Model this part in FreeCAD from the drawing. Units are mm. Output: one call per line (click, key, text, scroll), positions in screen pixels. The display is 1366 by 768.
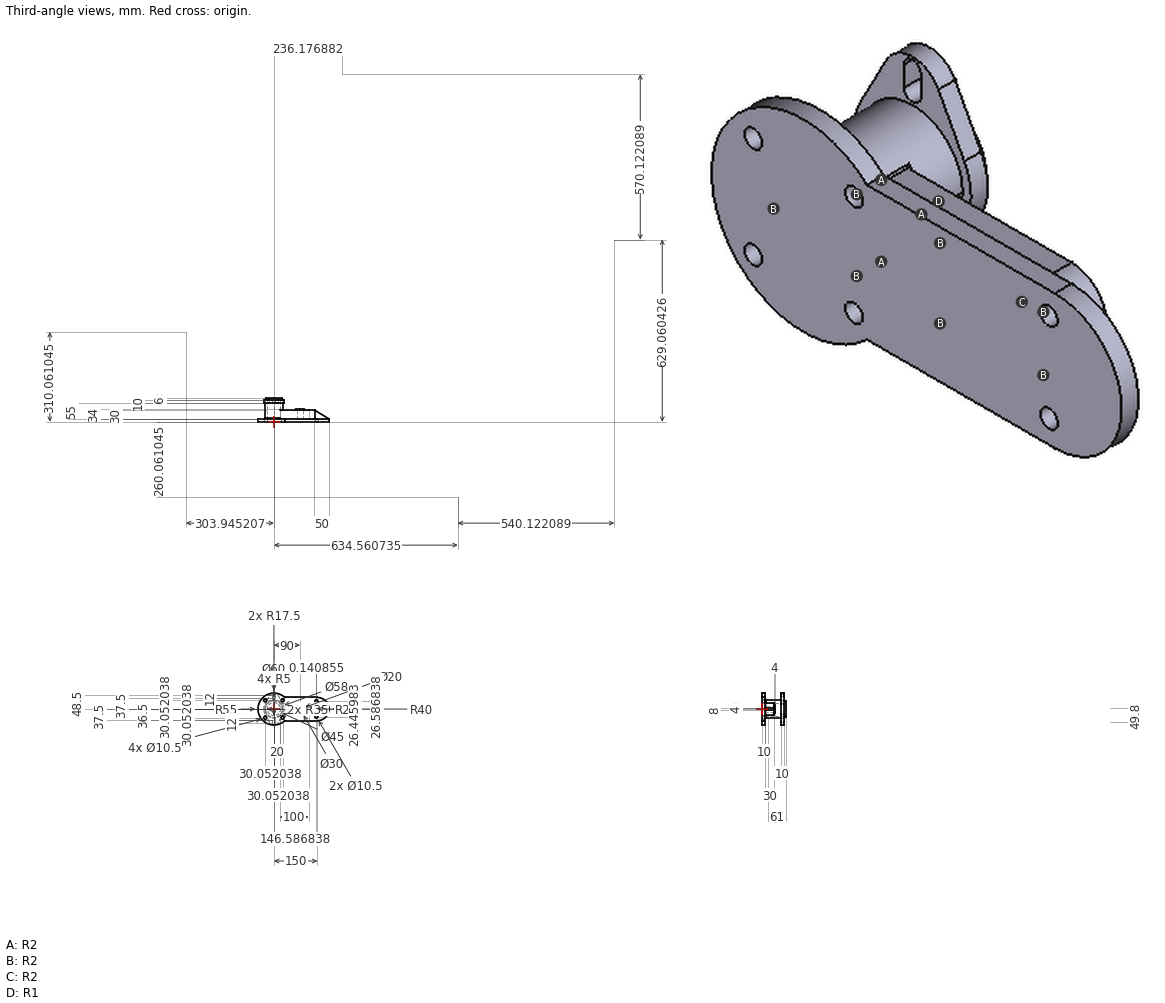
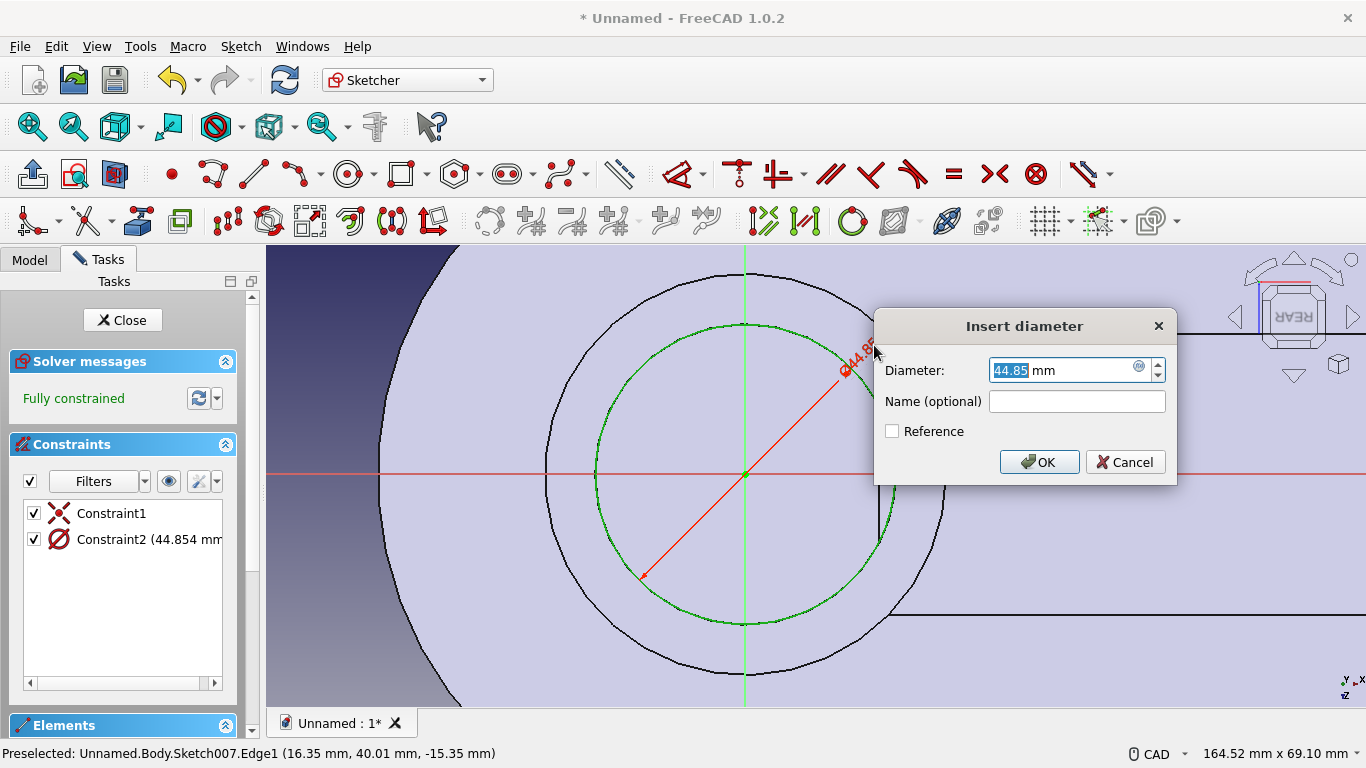
text(45)
key(Return)
key(Escape)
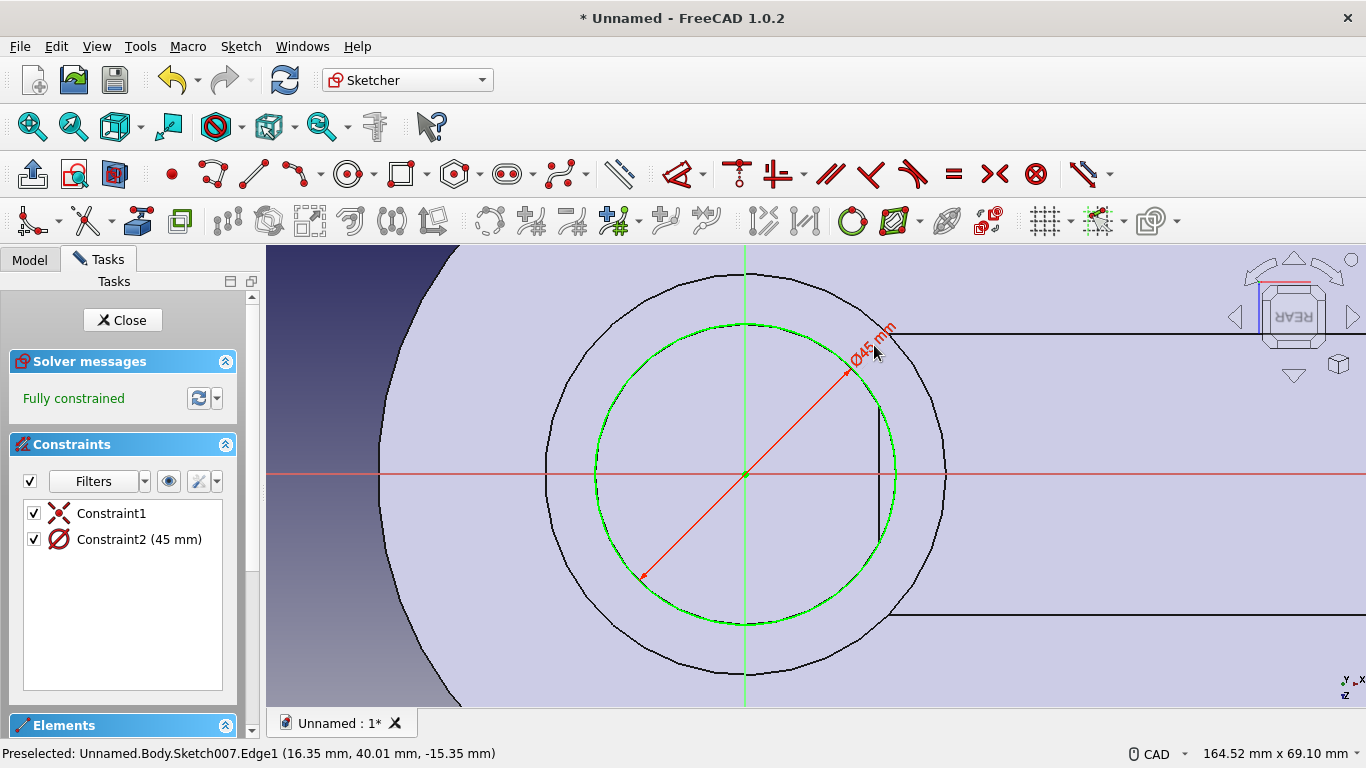
click(123, 320)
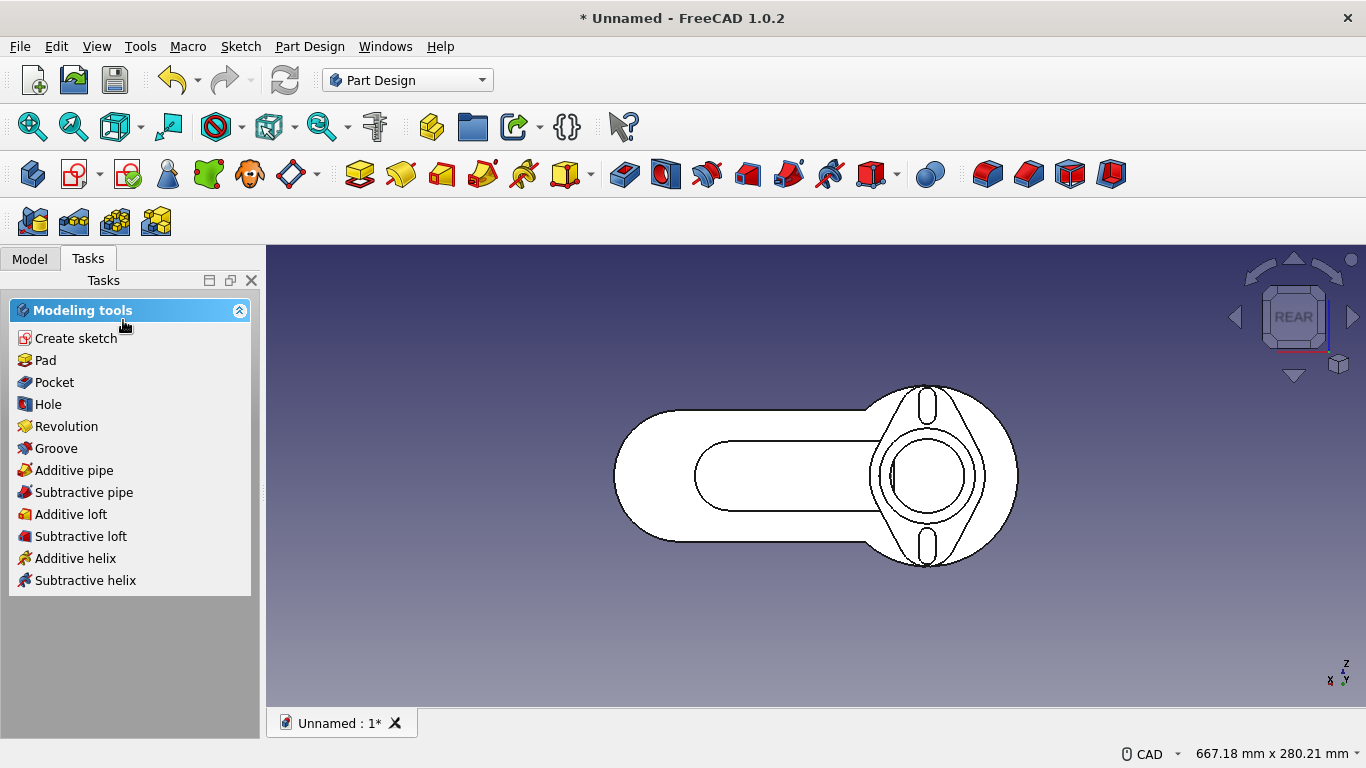
click(625, 174)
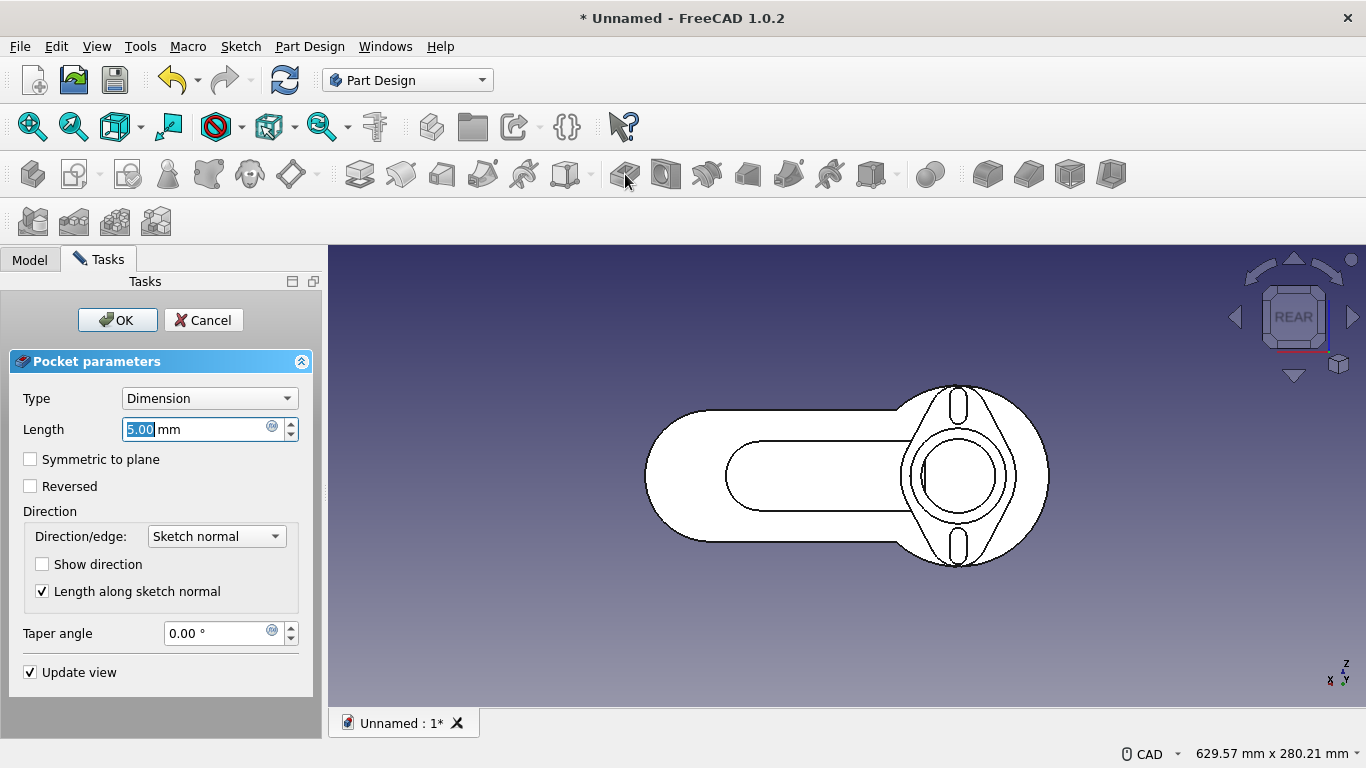
text(30)
key(Tab)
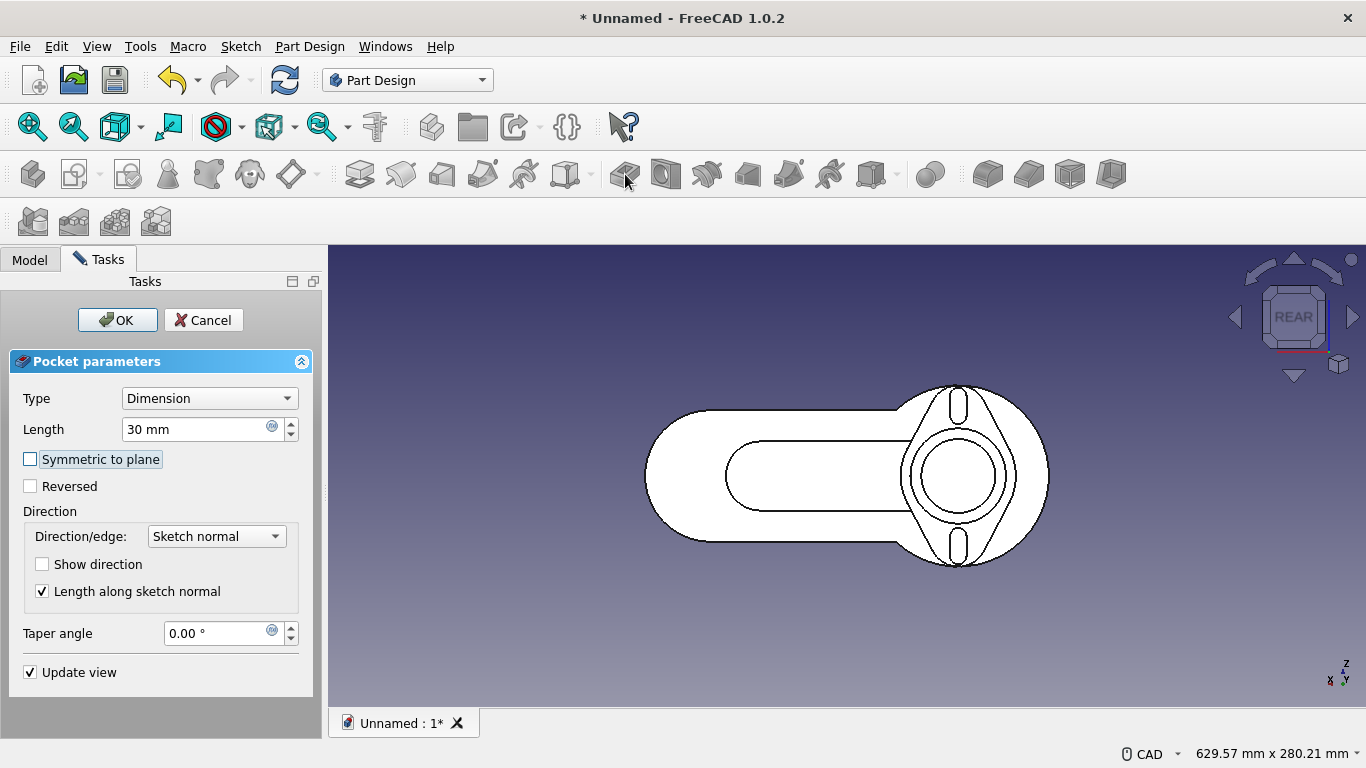
click(118, 320)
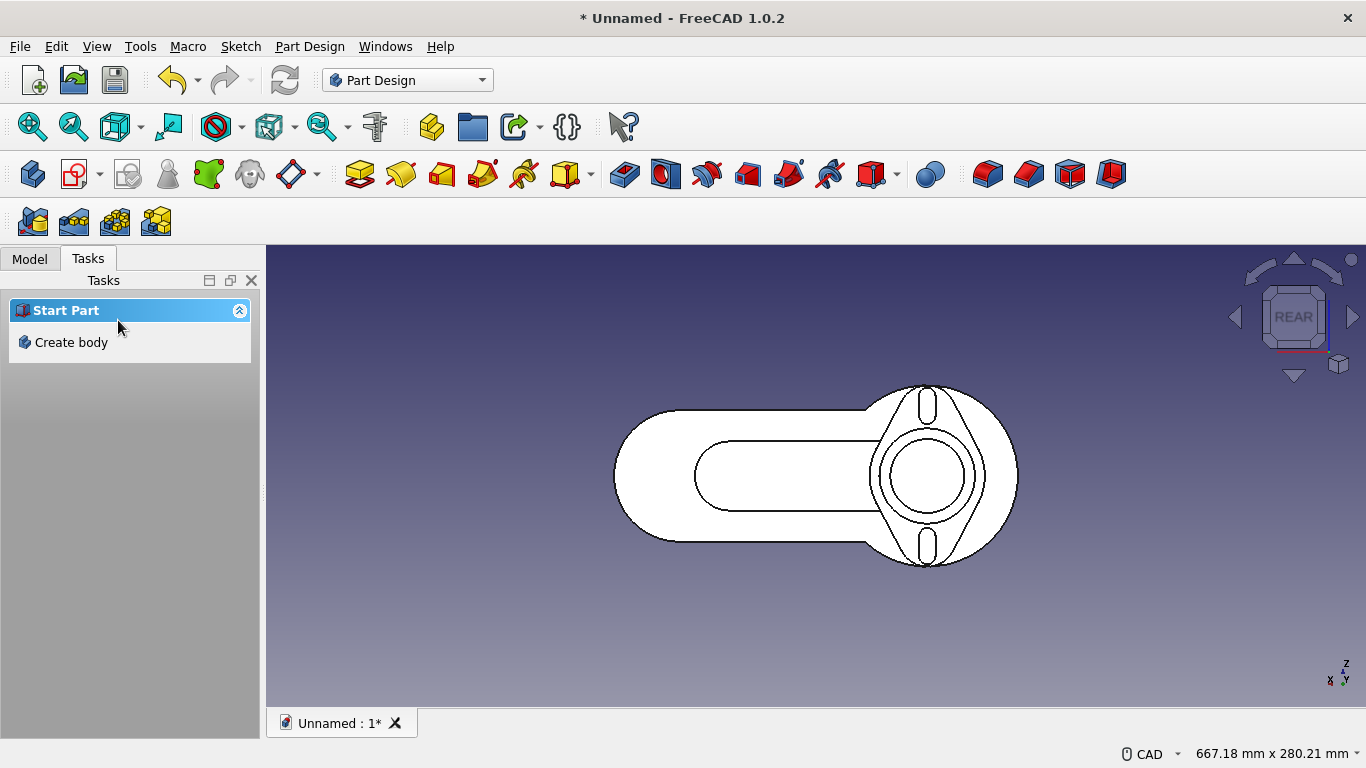
key(v)
key(f)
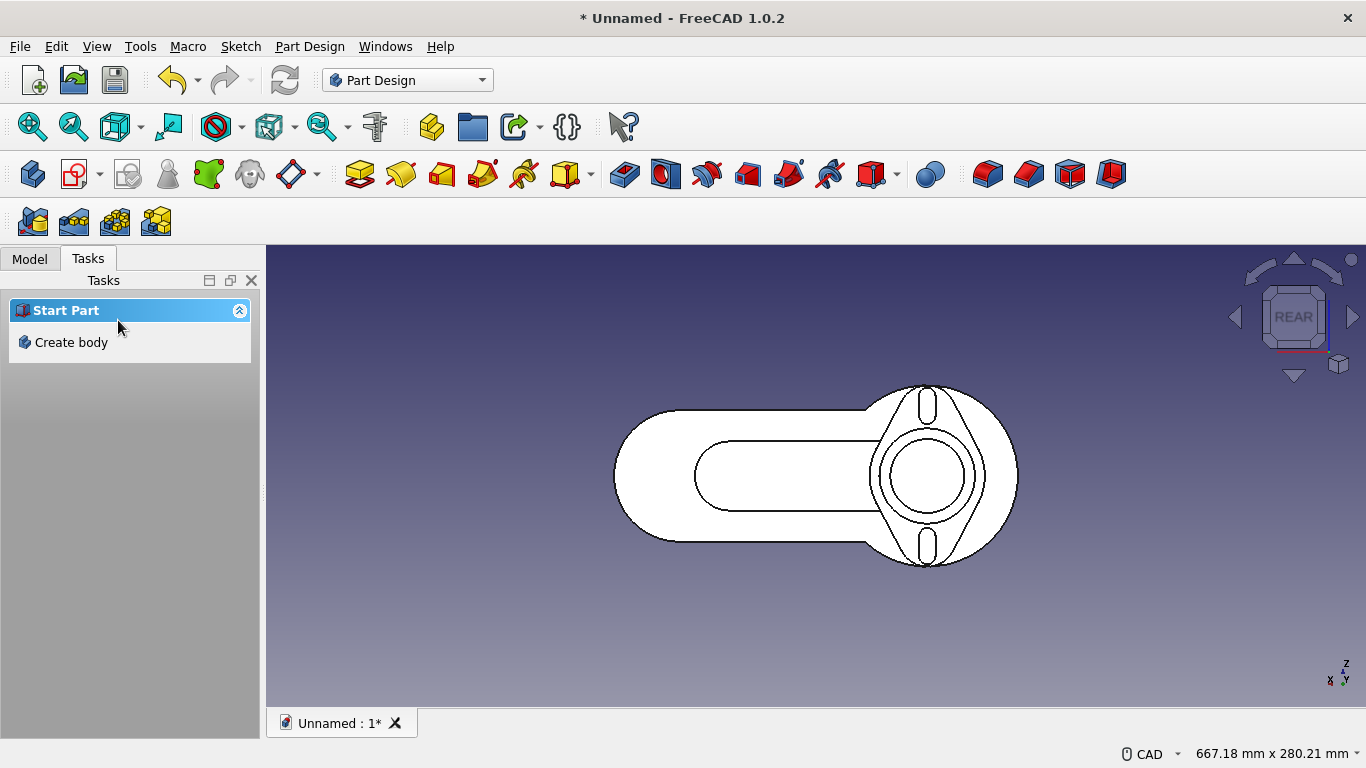
click(737, 475)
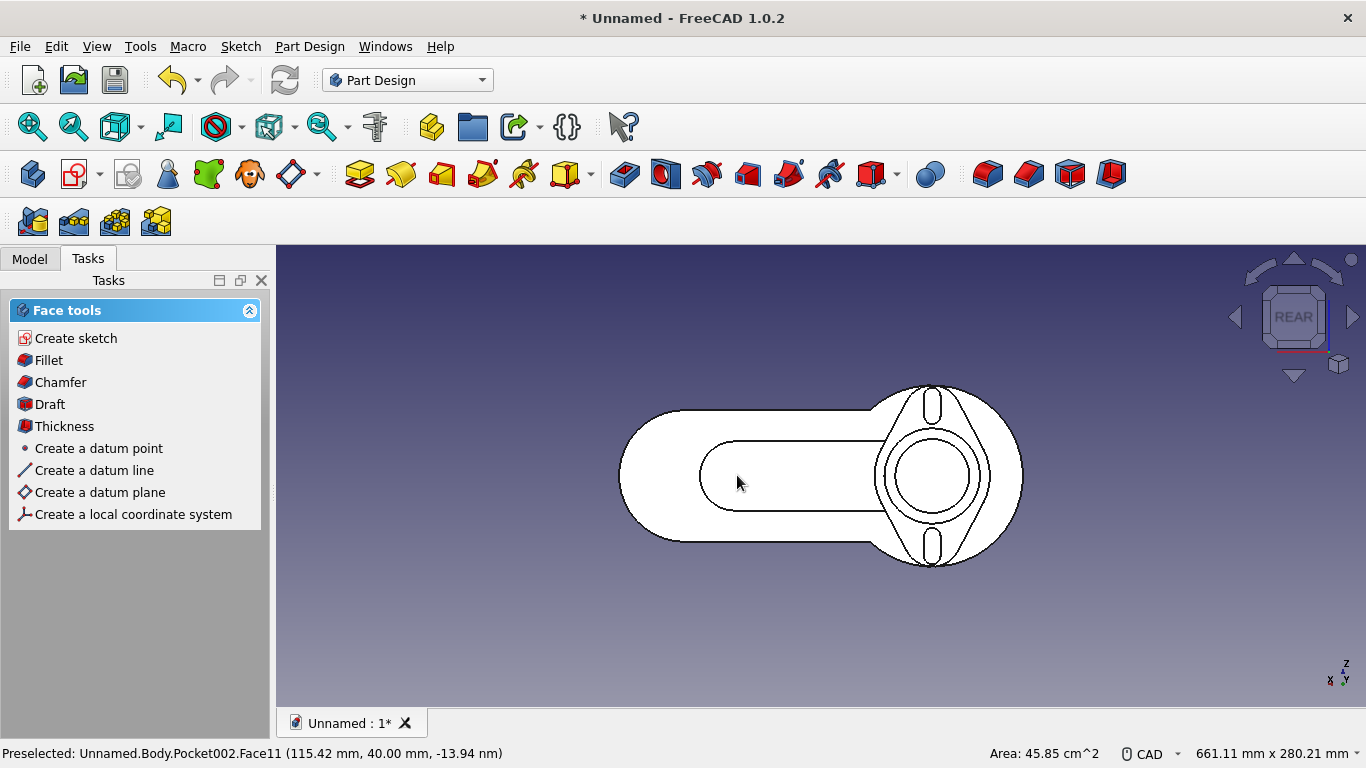
click(74, 174)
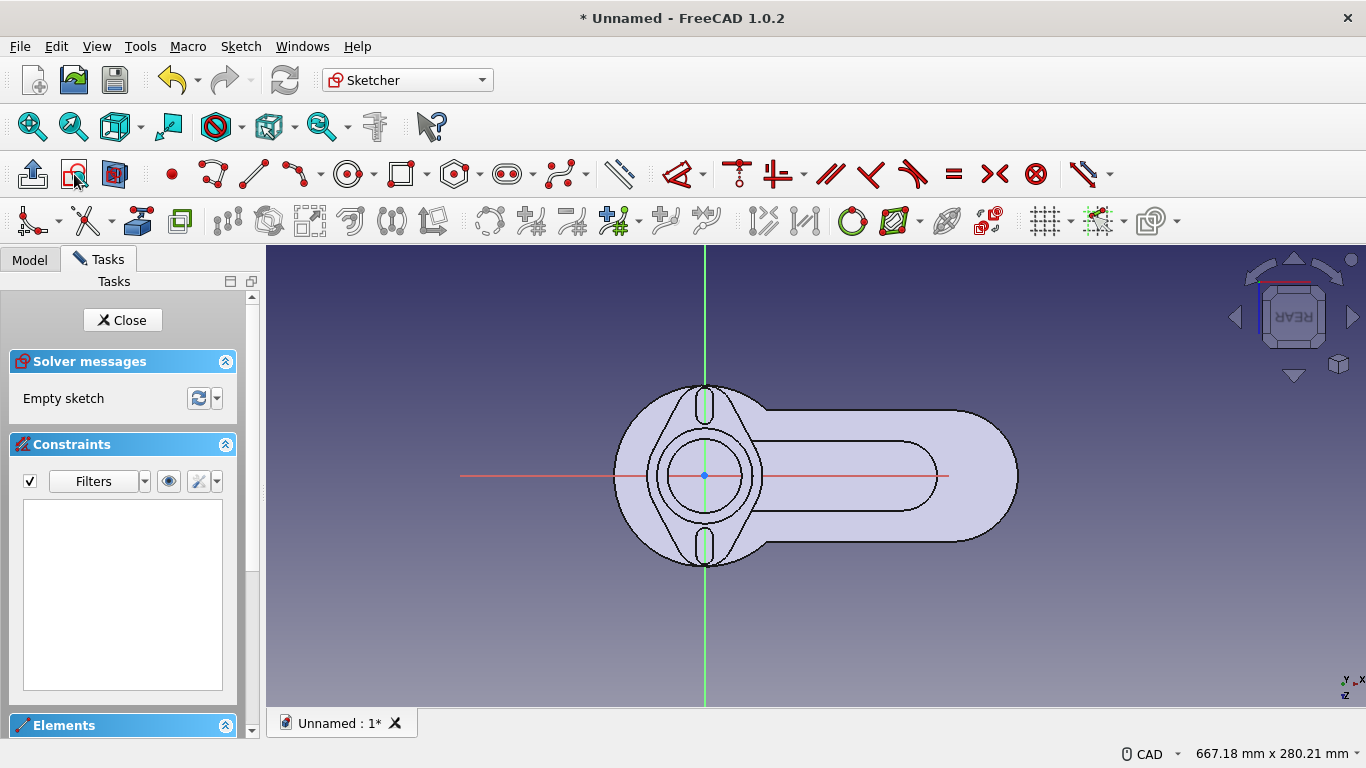
key(q)
key(s)